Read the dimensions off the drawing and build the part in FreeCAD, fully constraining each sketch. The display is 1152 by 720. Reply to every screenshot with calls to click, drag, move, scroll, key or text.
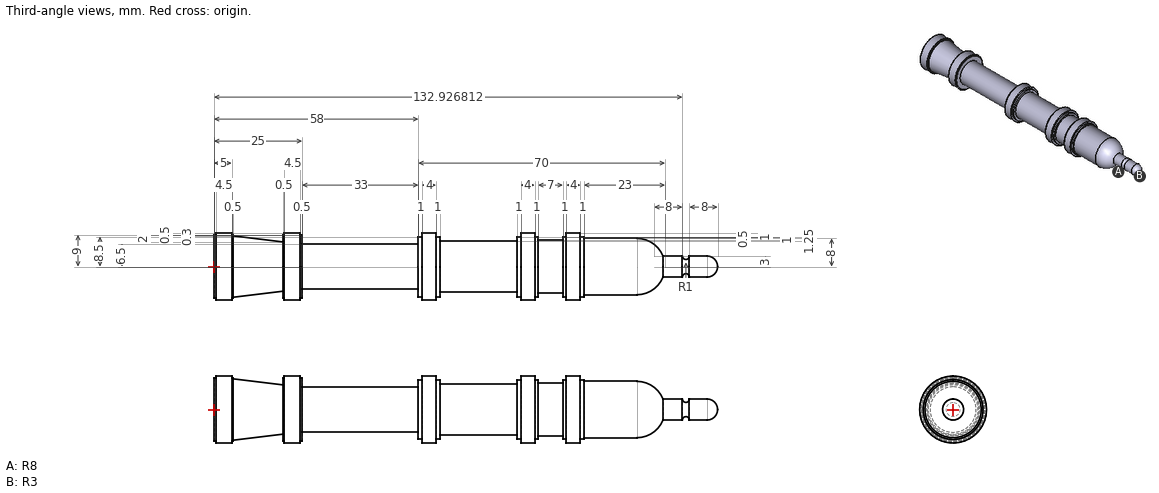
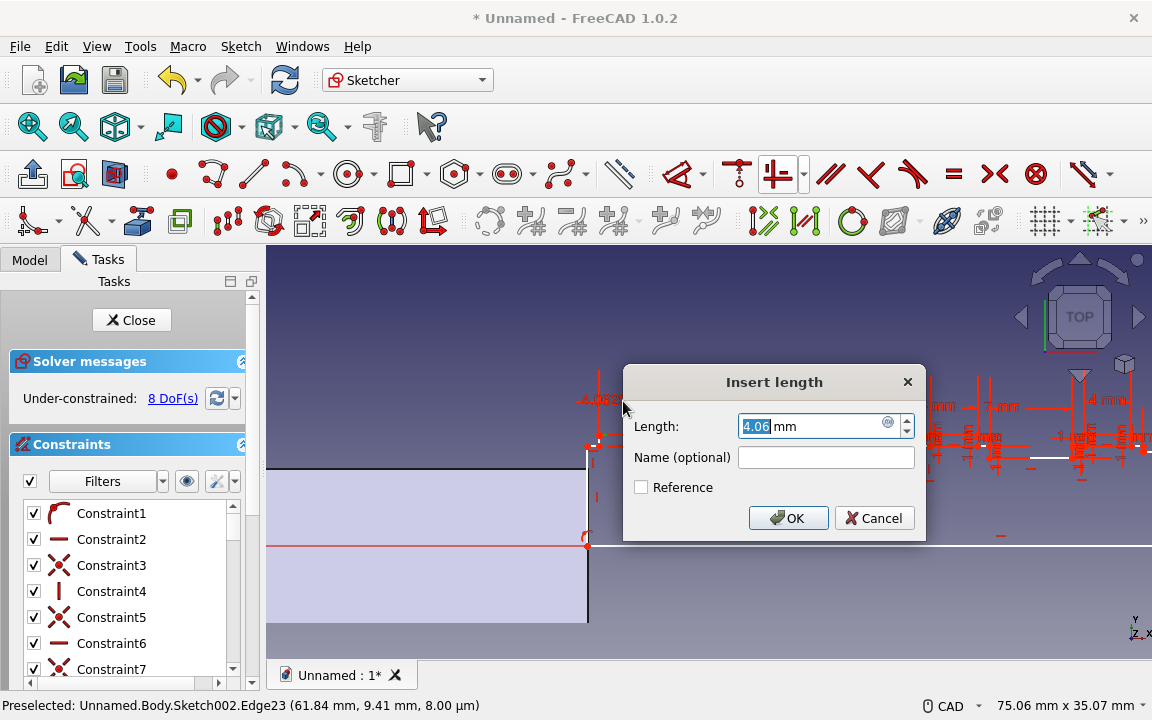
text(4)
key(Return)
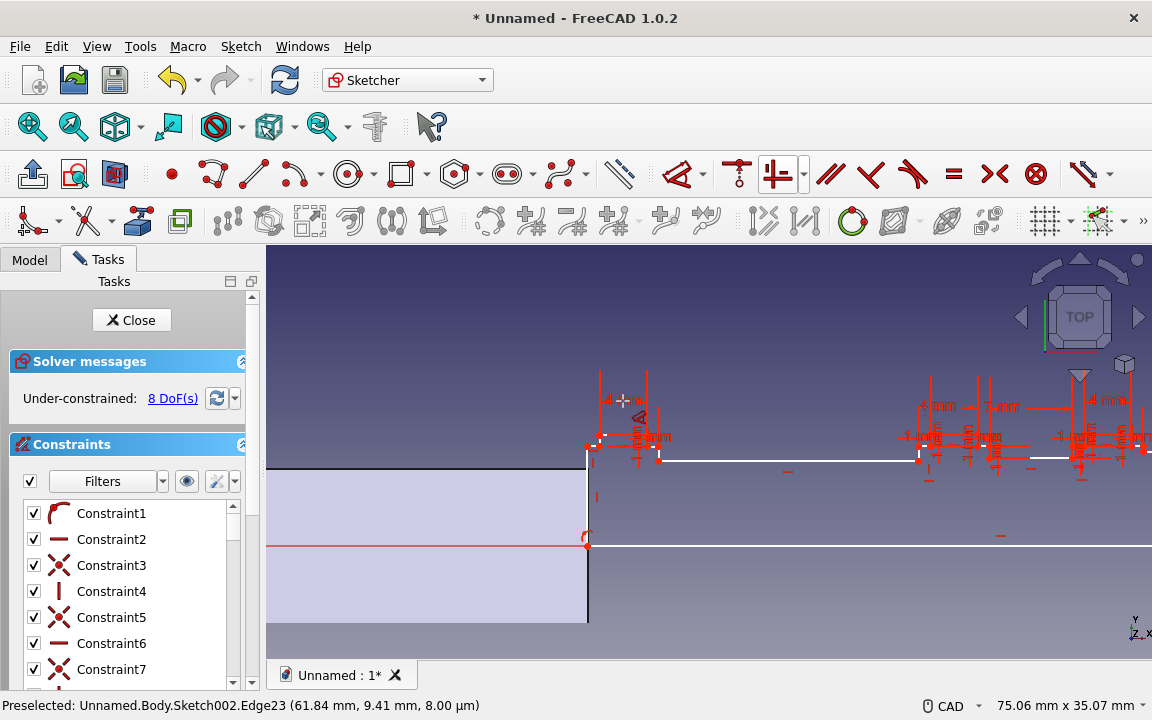
scroll(600, 441, up, 7)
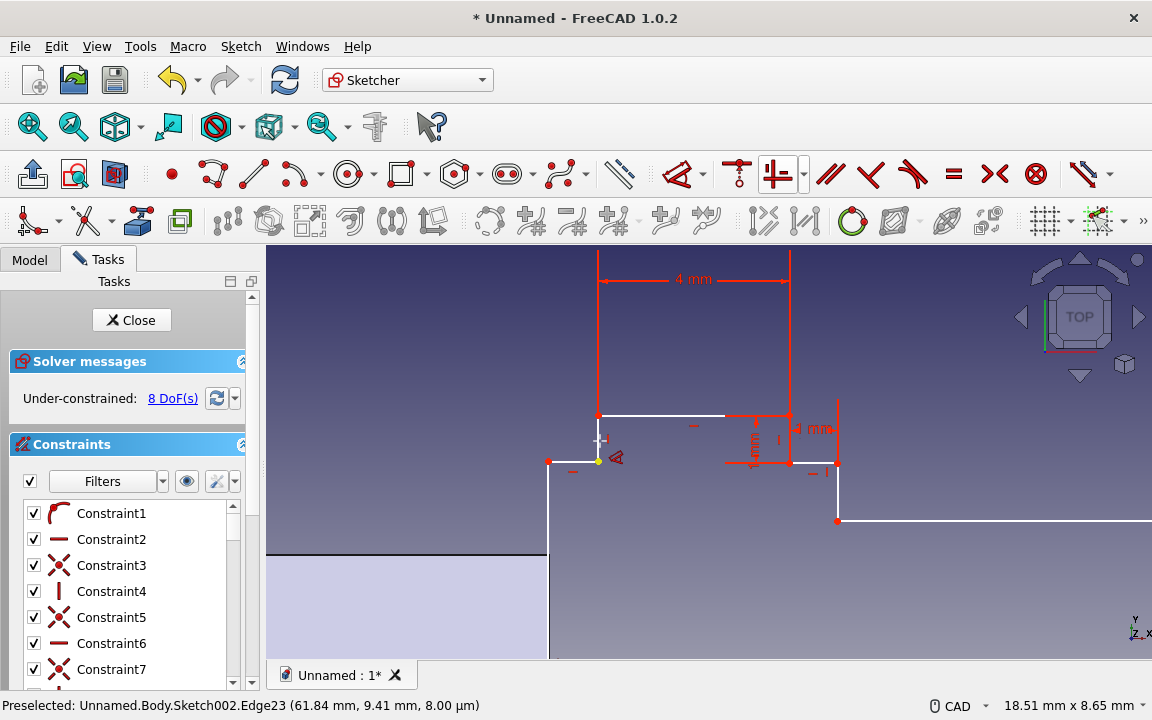
click(598, 439)
click(564, 439)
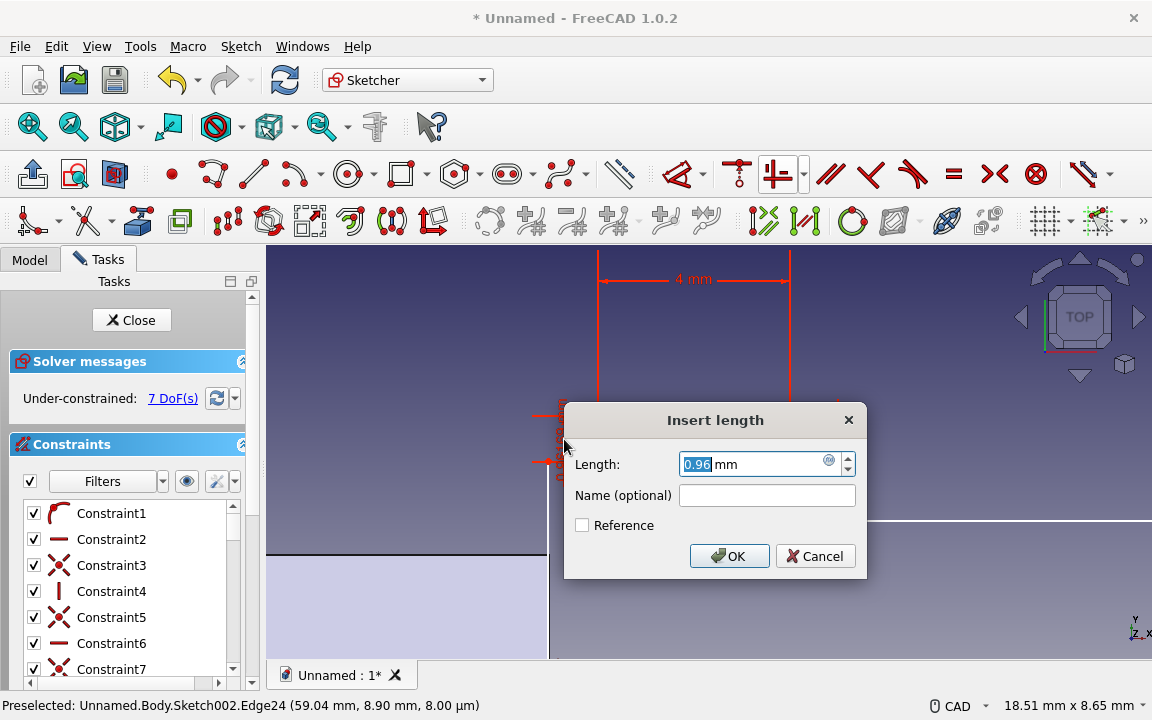
text(1)
key(Return)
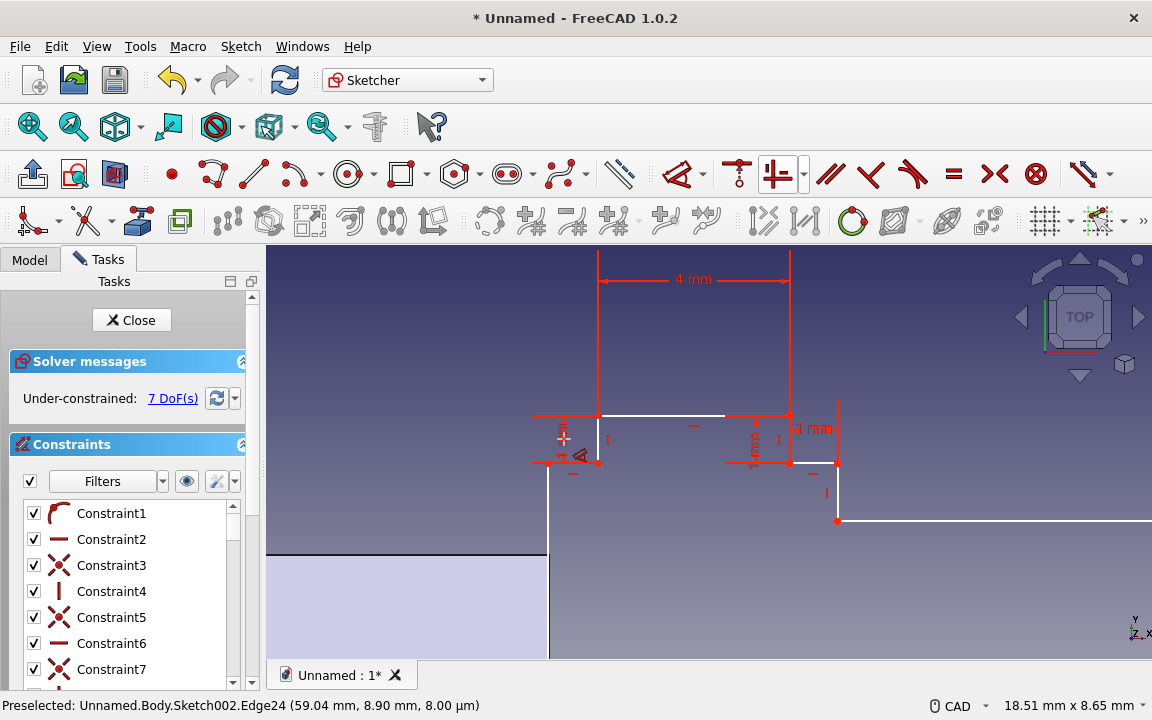
click(583, 463)
click(573, 497)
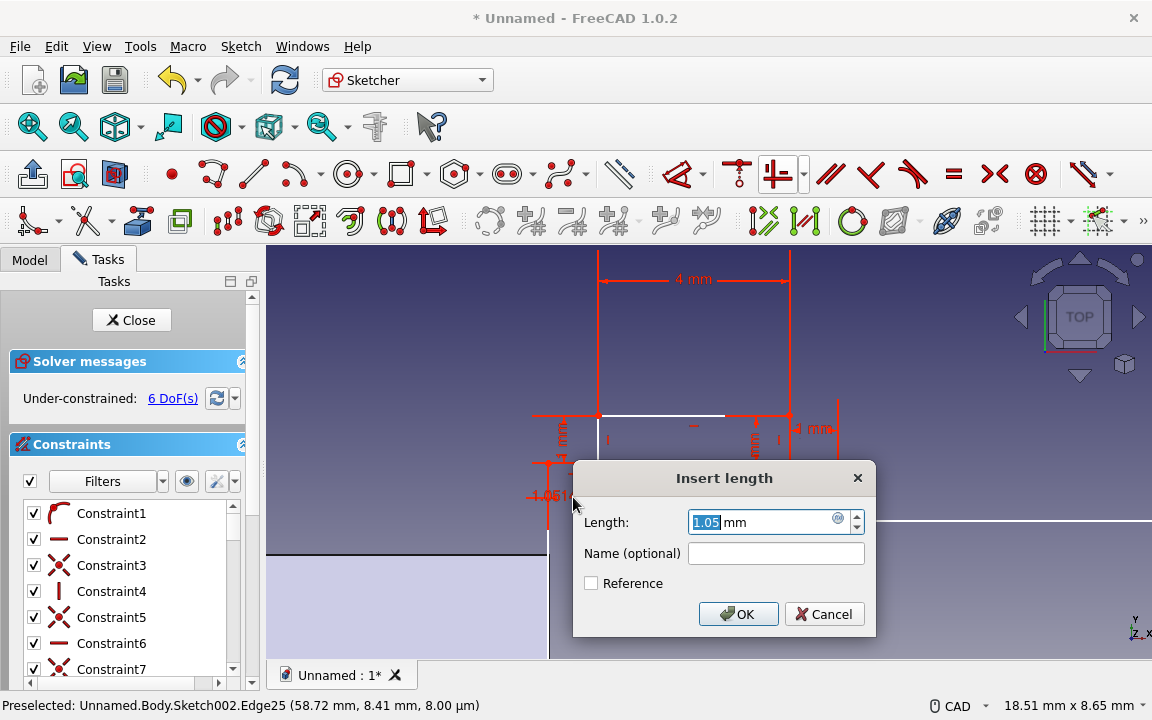
text(1)
key(Return)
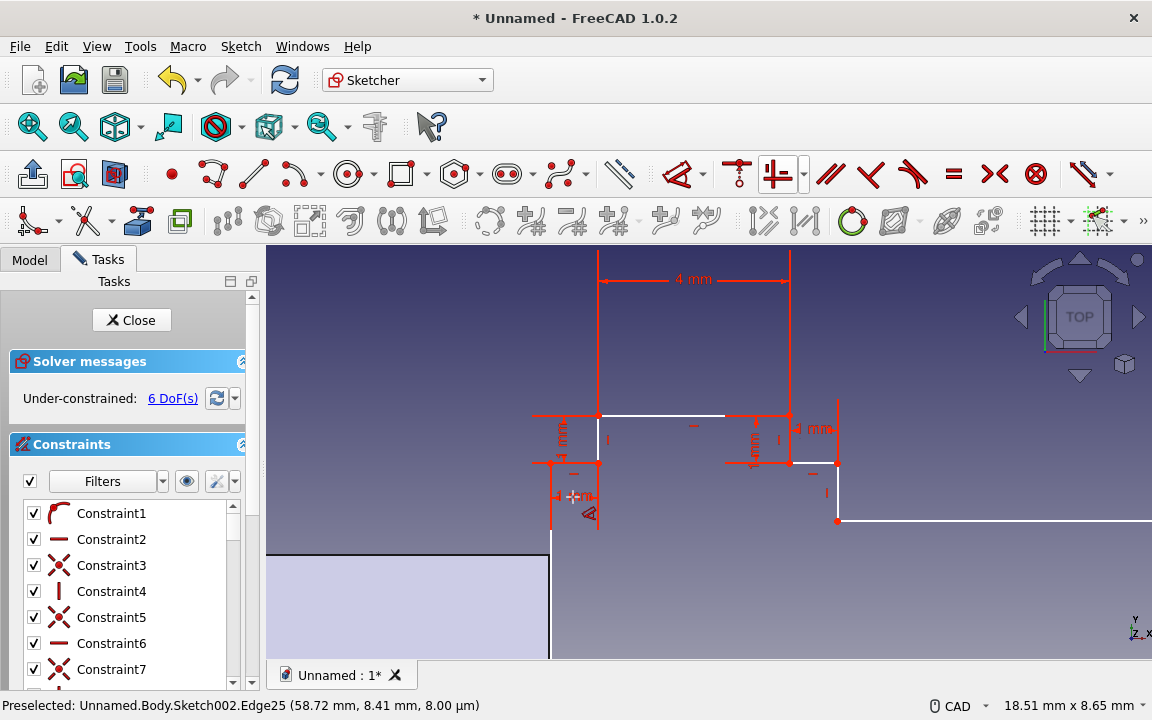
scroll(625, 437, down, 13)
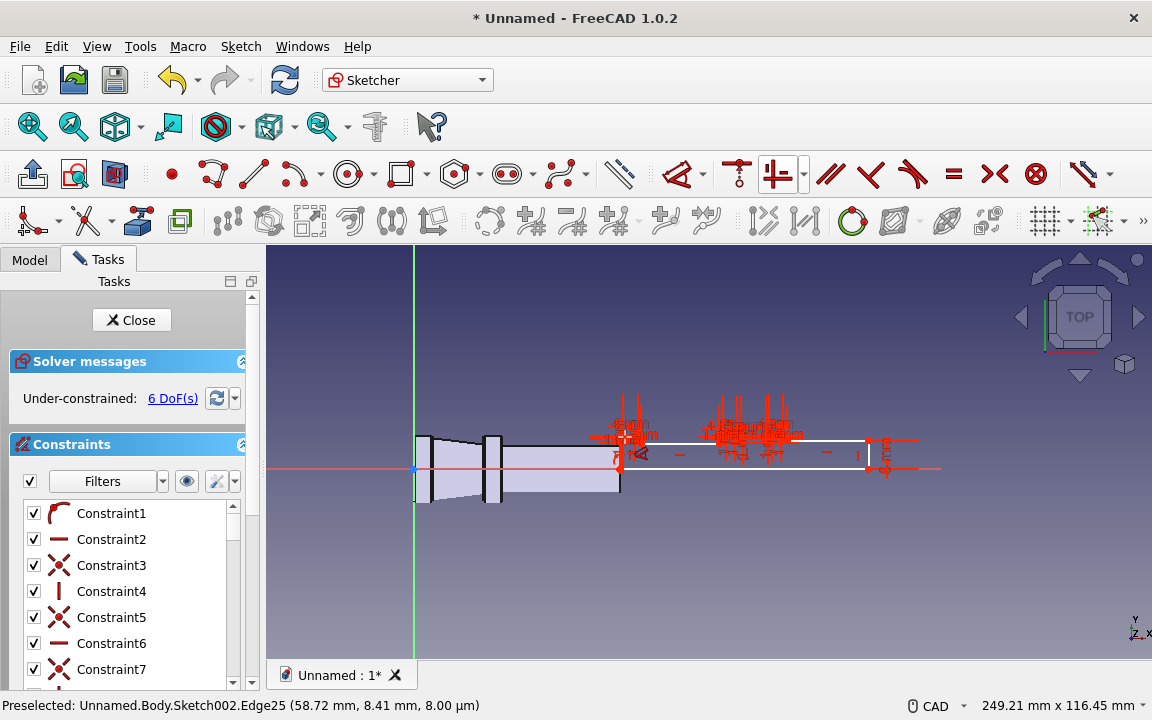
click(695, 469)
click(744, 503)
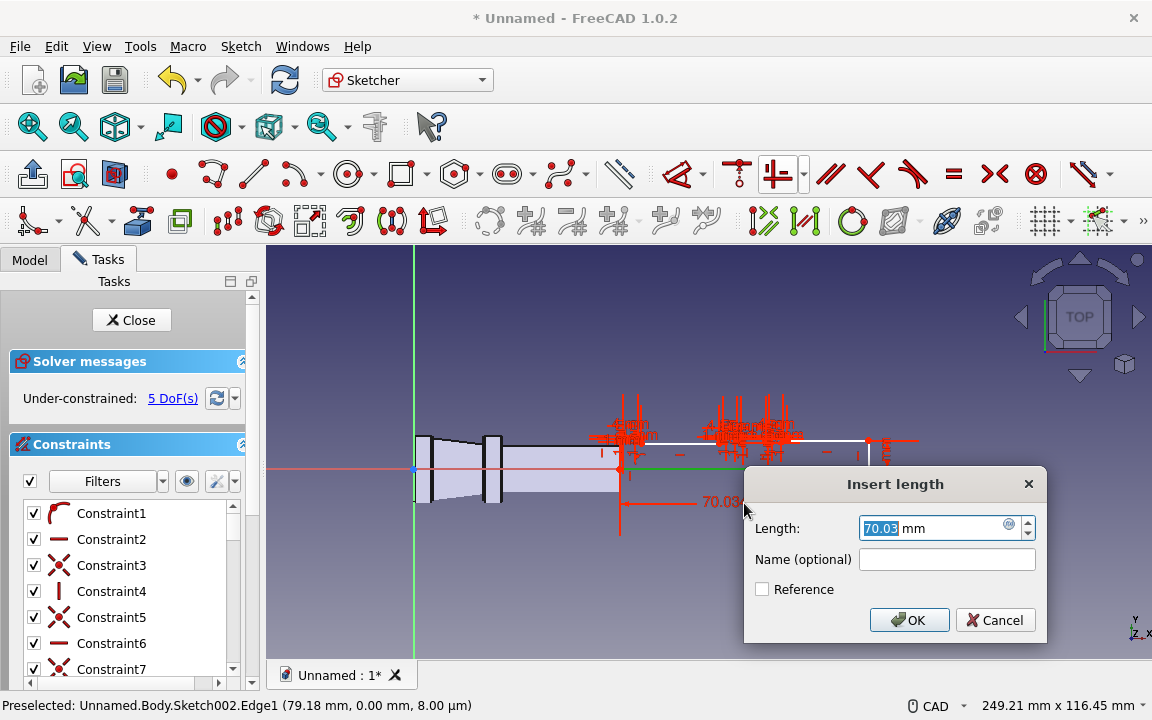
text(70)
key(Return)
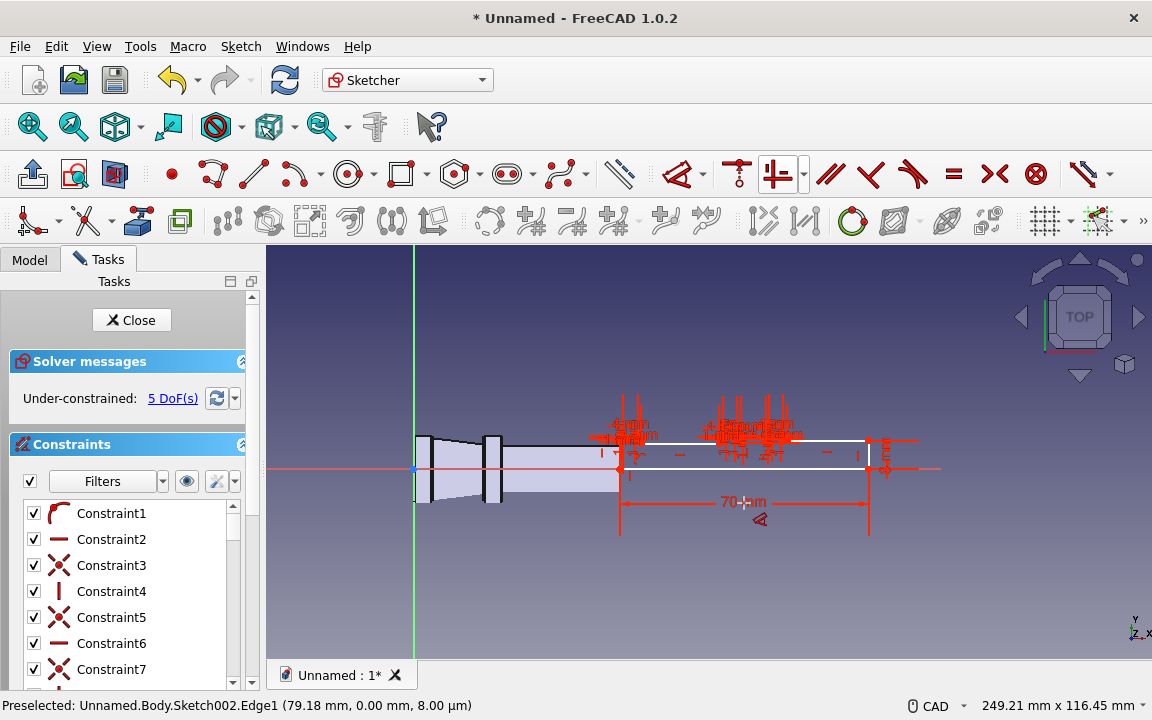
click(844, 441)
click(847, 407)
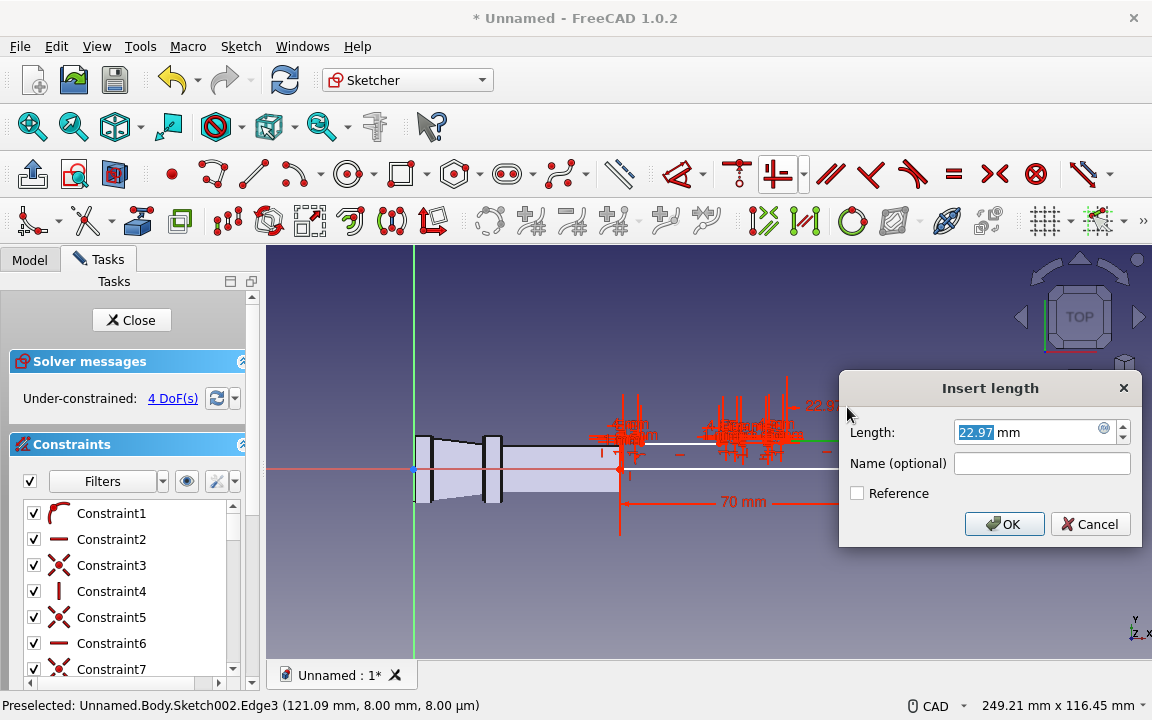
text(23)
key(Return)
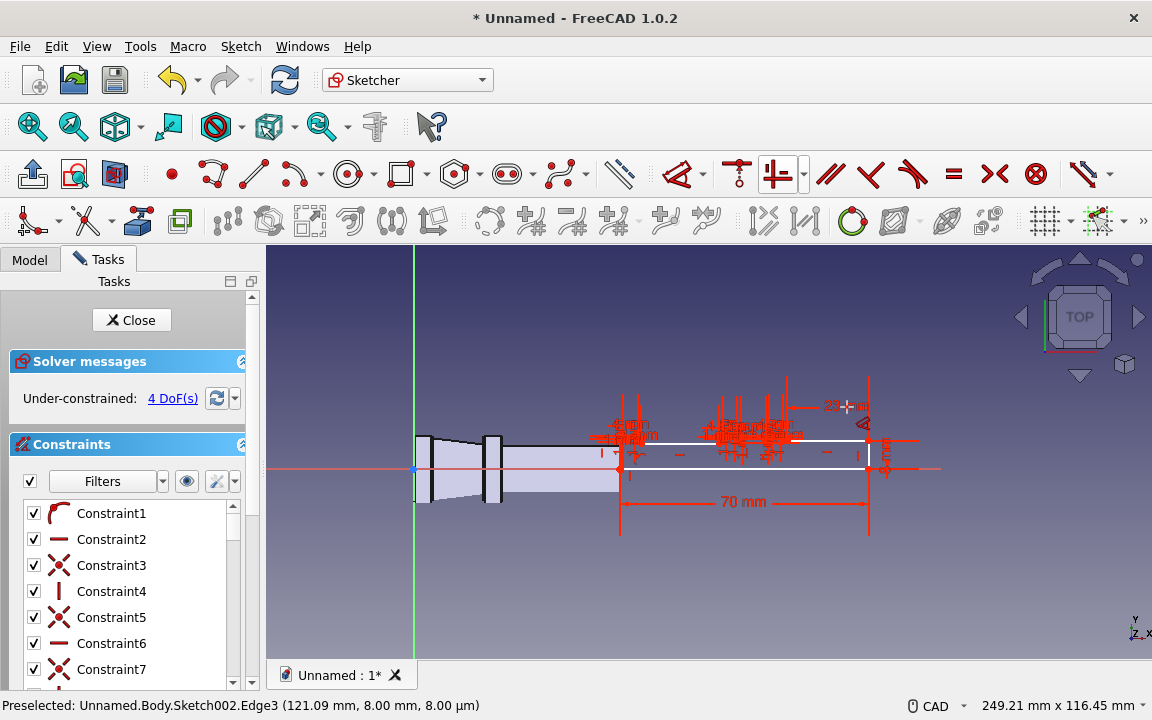
scroll(787, 440, up, 16)